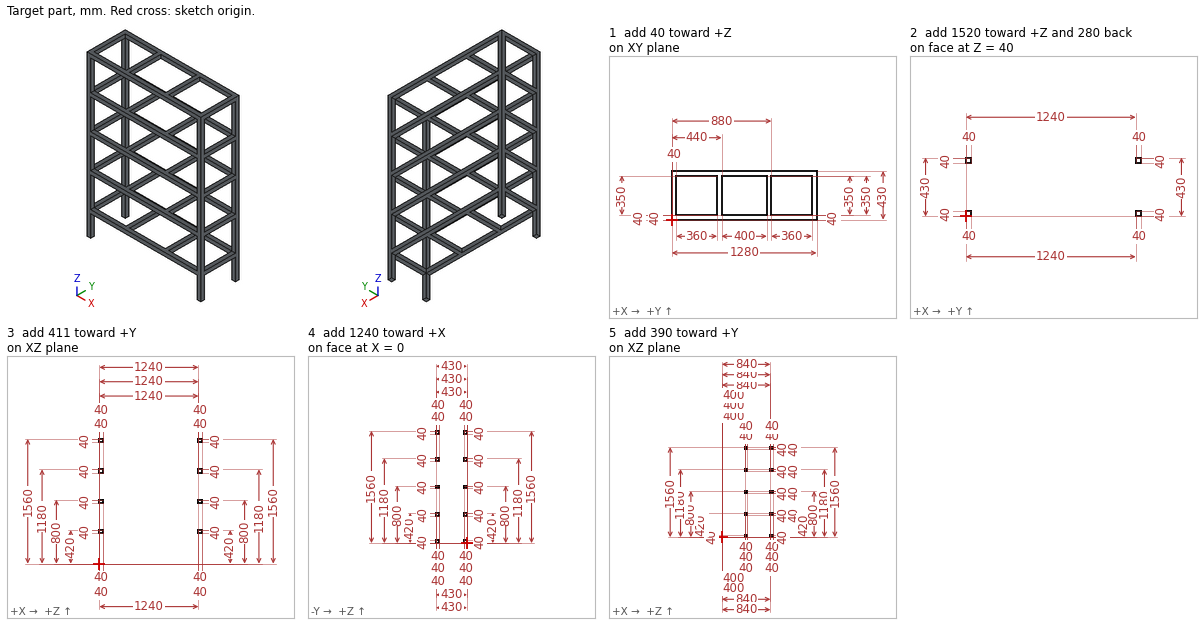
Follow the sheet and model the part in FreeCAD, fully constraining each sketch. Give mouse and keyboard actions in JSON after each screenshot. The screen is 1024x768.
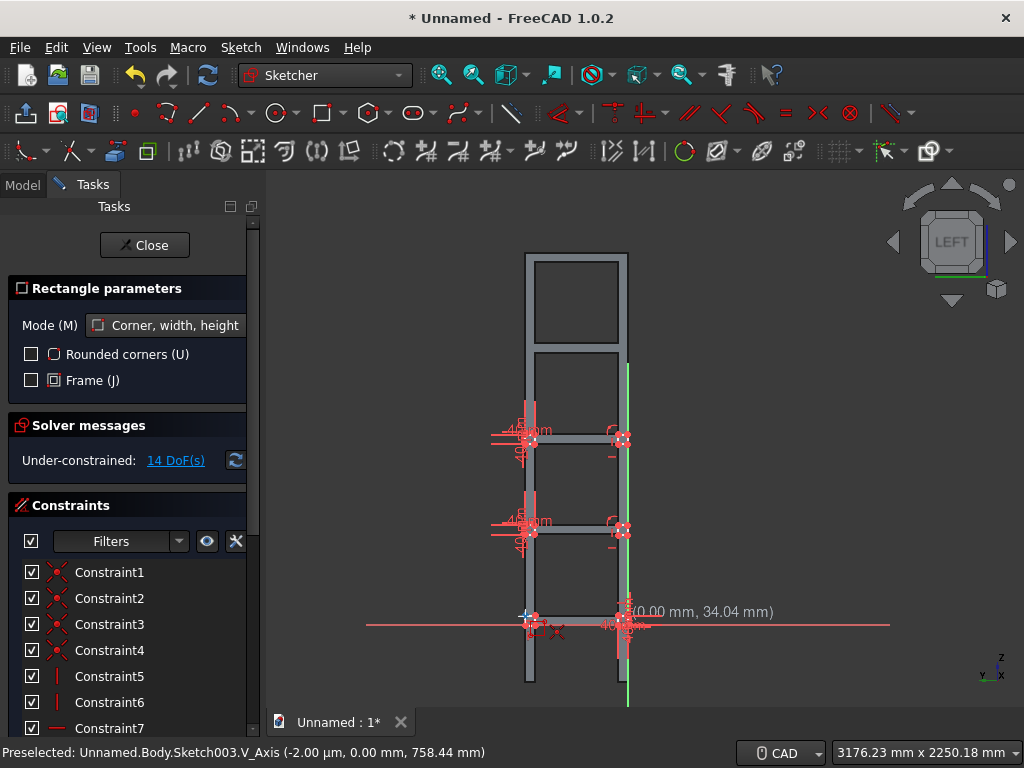
{"action": "scroll", "coordinate": [618, 343], "scroll_direction": "up", "scroll_amount": 3}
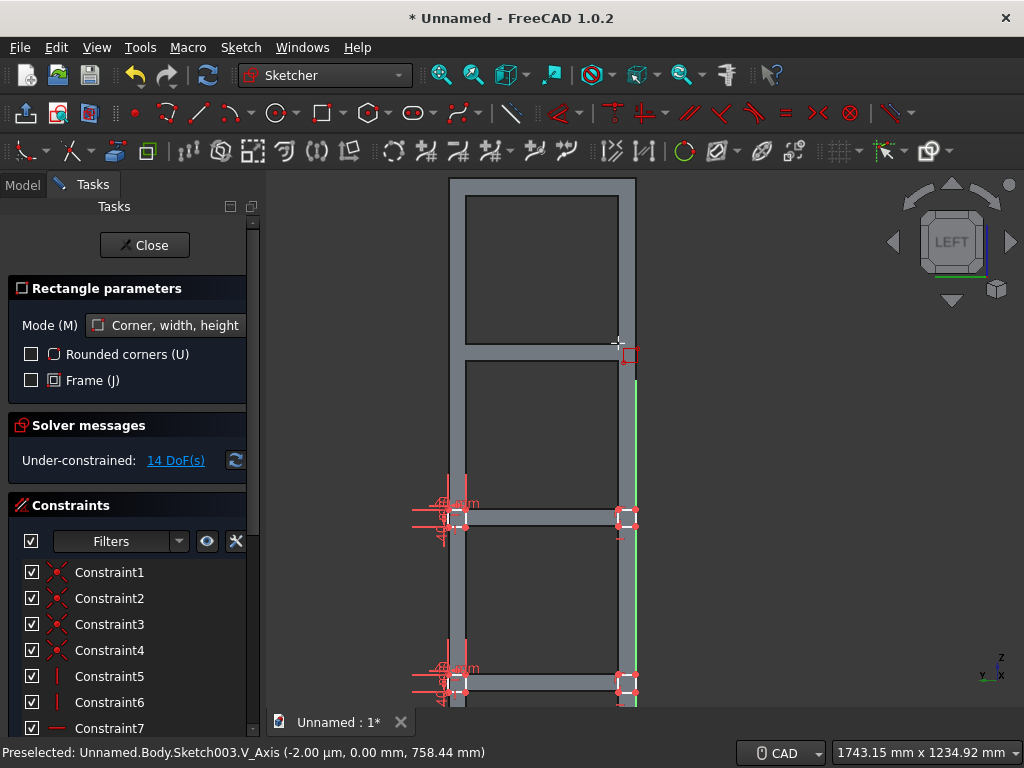
{"action": "left_click", "coordinate": [618, 344]}
{"action": "left_click", "coordinate": [636, 361]}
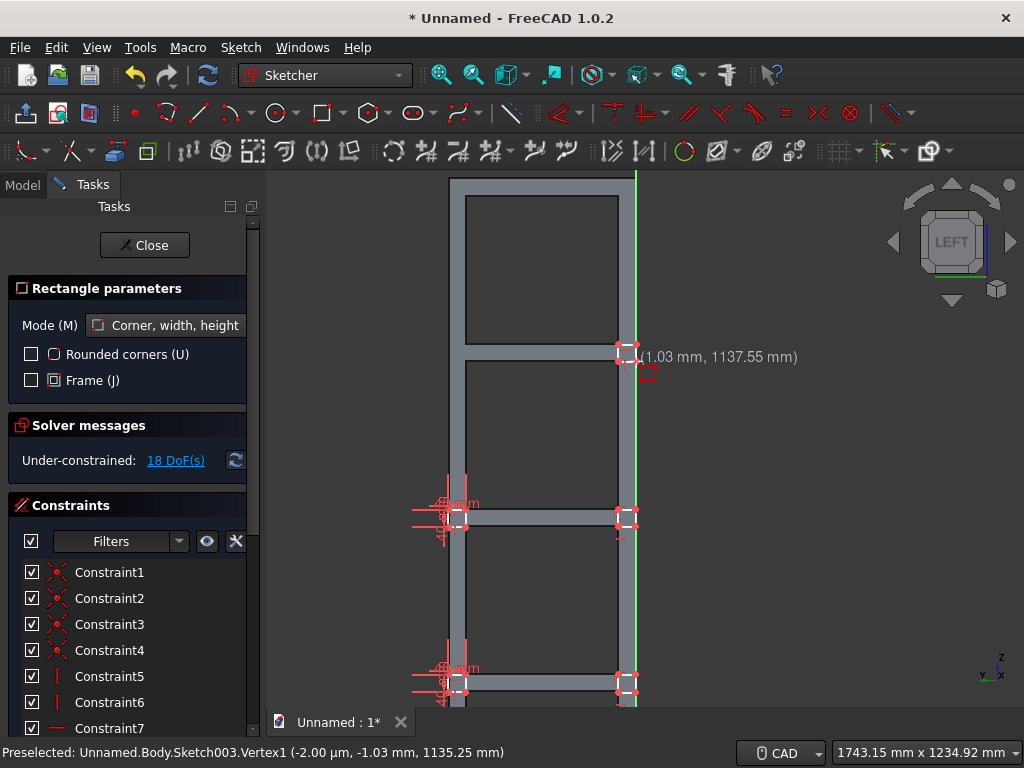
{"action": "left_click", "coordinate": [449, 344]}
{"action": "mouse_move", "coordinate": [466, 361]}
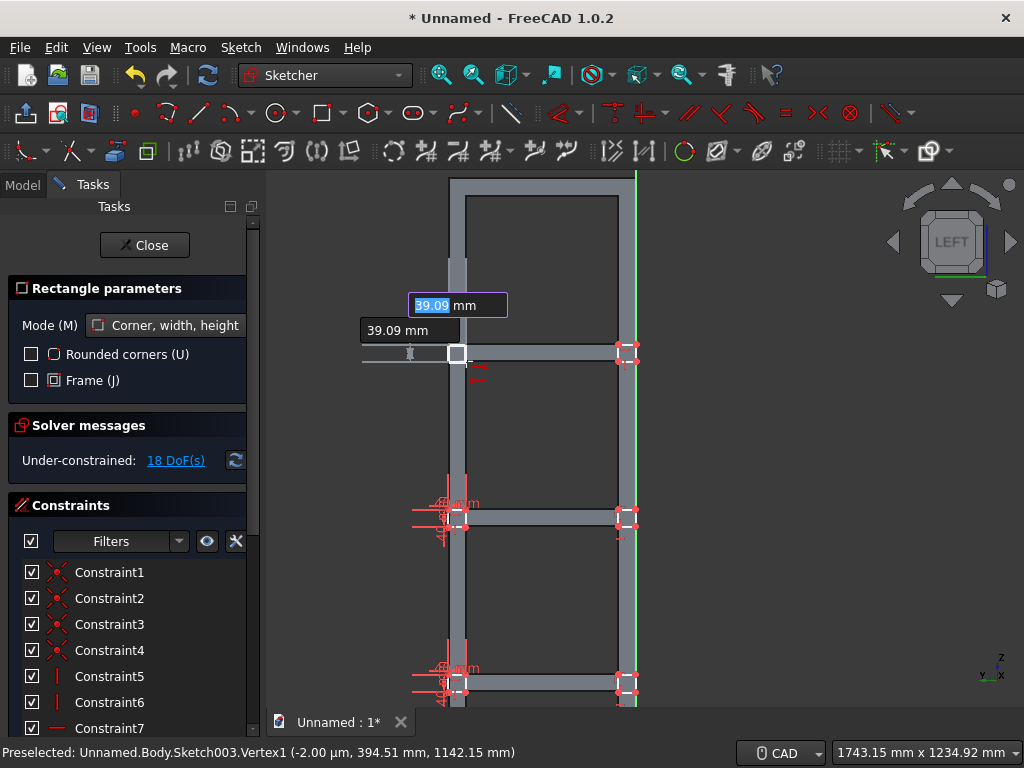
{"action": "type", "text": "40"}
{"action": "key", "text": "Tab"}
{"action": "type", "text": "40"}
{"action": "key", "text": "Return"}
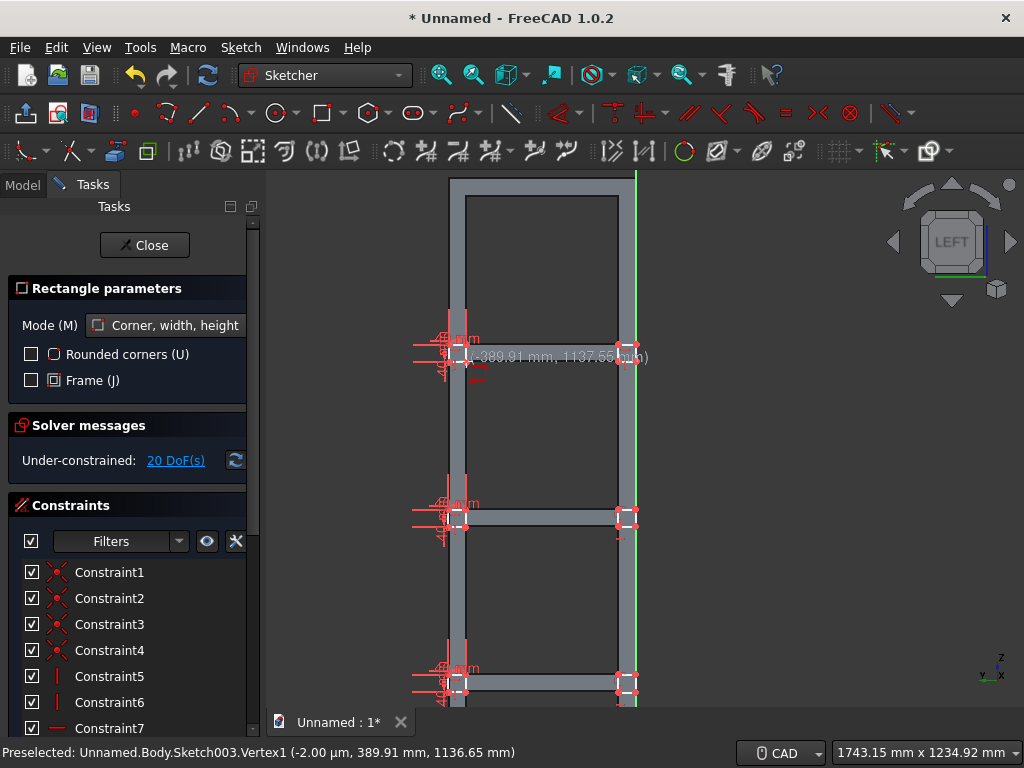
{"action": "scroll", "coordinate": [618, 342], "scroll_direction": "down", "scroll_amount": 3}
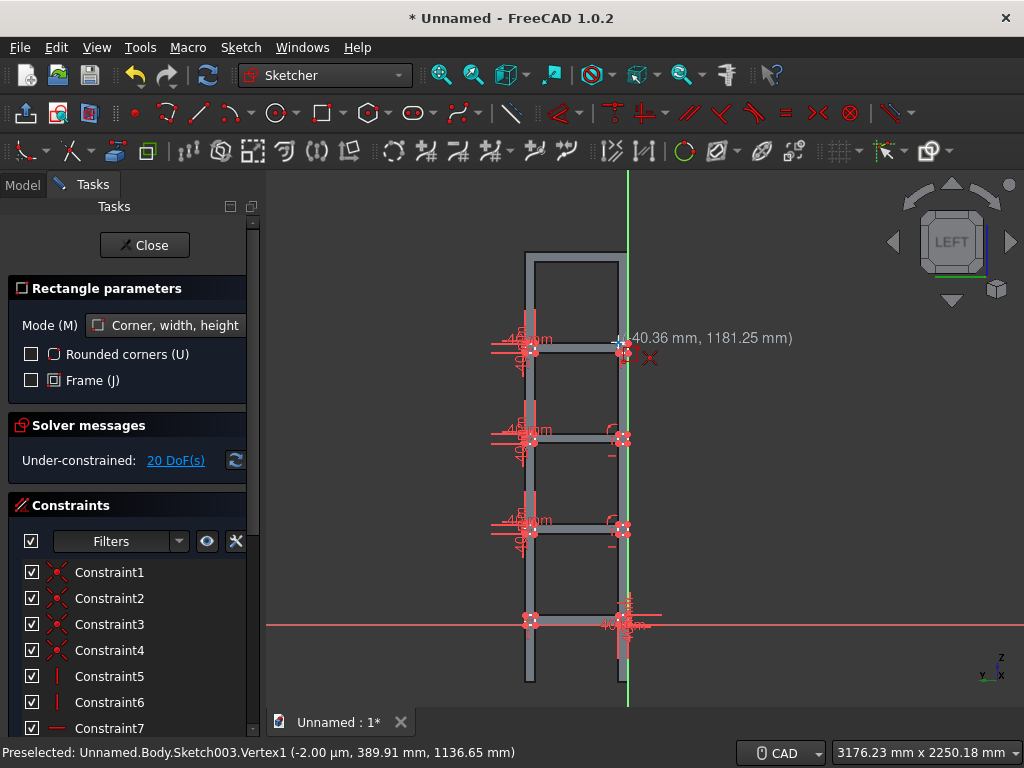
{"action": "scroll", "coordinate": [525, 252], "scroll_direction": "up", "scroll_amount": 3}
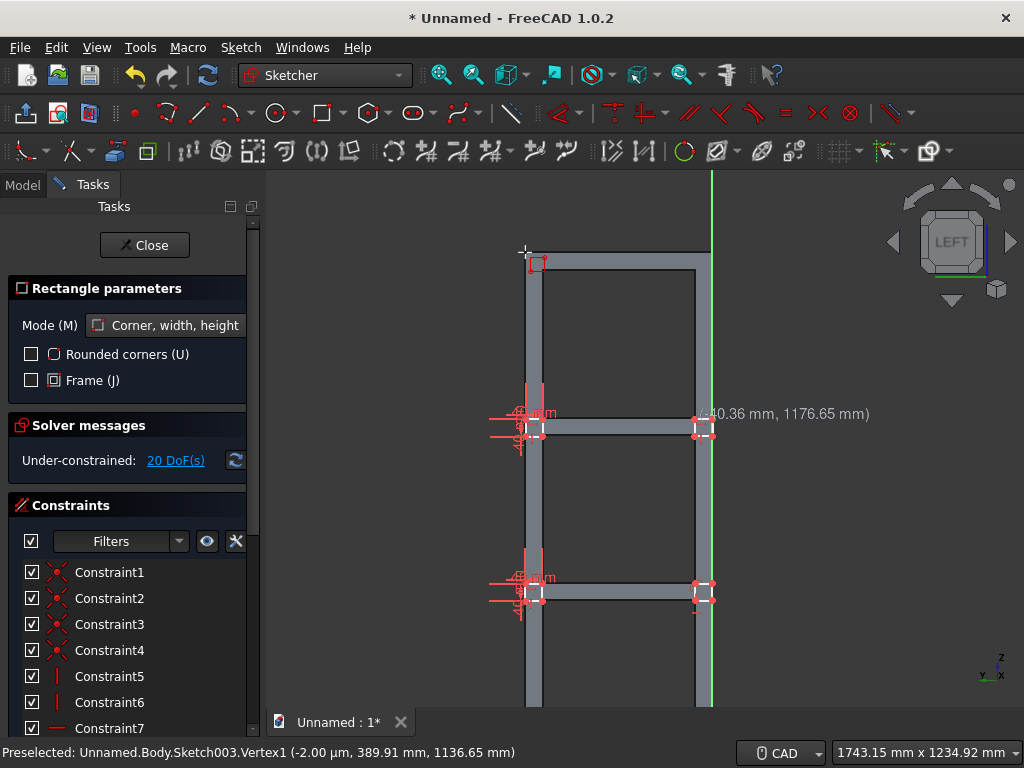
{"action": "left_click", "coordinate": [525, 252]}
{"action": "mouse_move", "coordinate": [543, 270]}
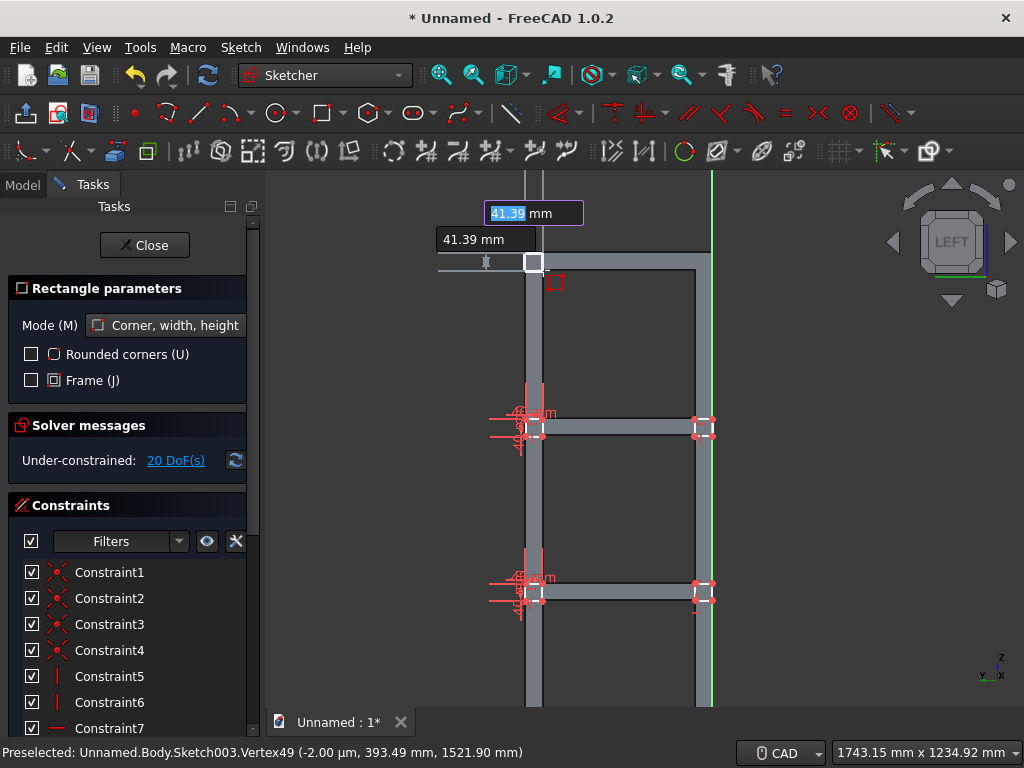
{"action": "type", "text": "40"}
{"action": "key", "text": "Tab"}
{"action": "type", "text": "40"}
{"action": "key", "text": "Return"}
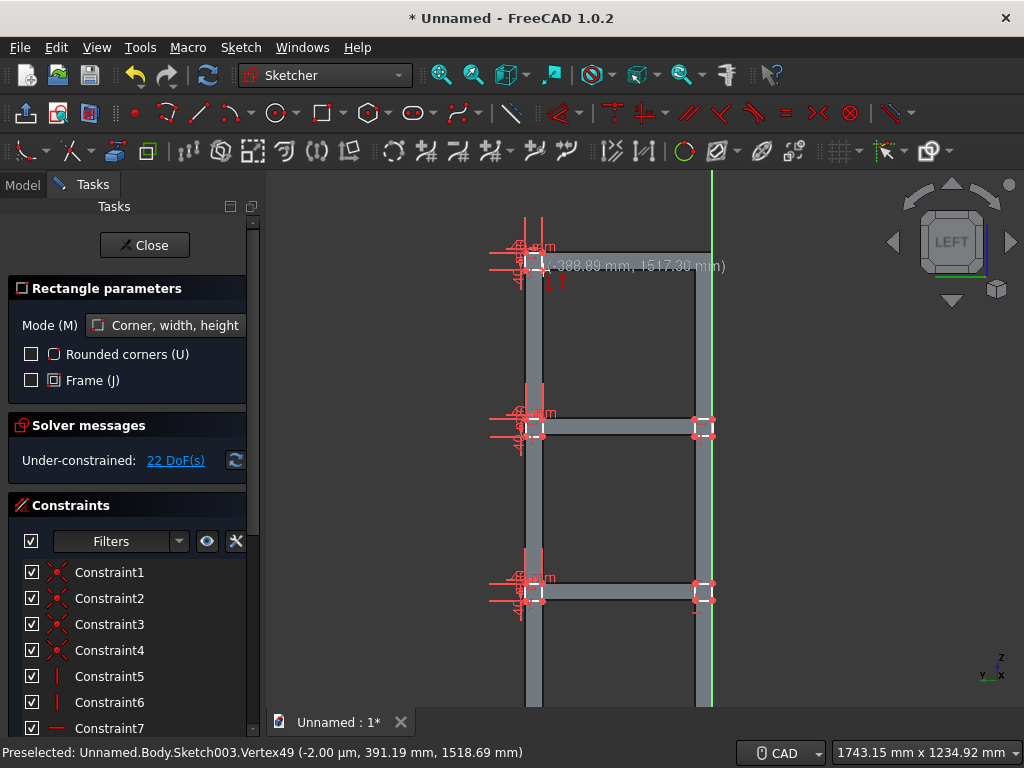
{"action": "left_click", "coordinate": [695, 252]}
{"action": "left_click", "coordinate": [712, 270]}
{"action": "key", "text": "Escape"}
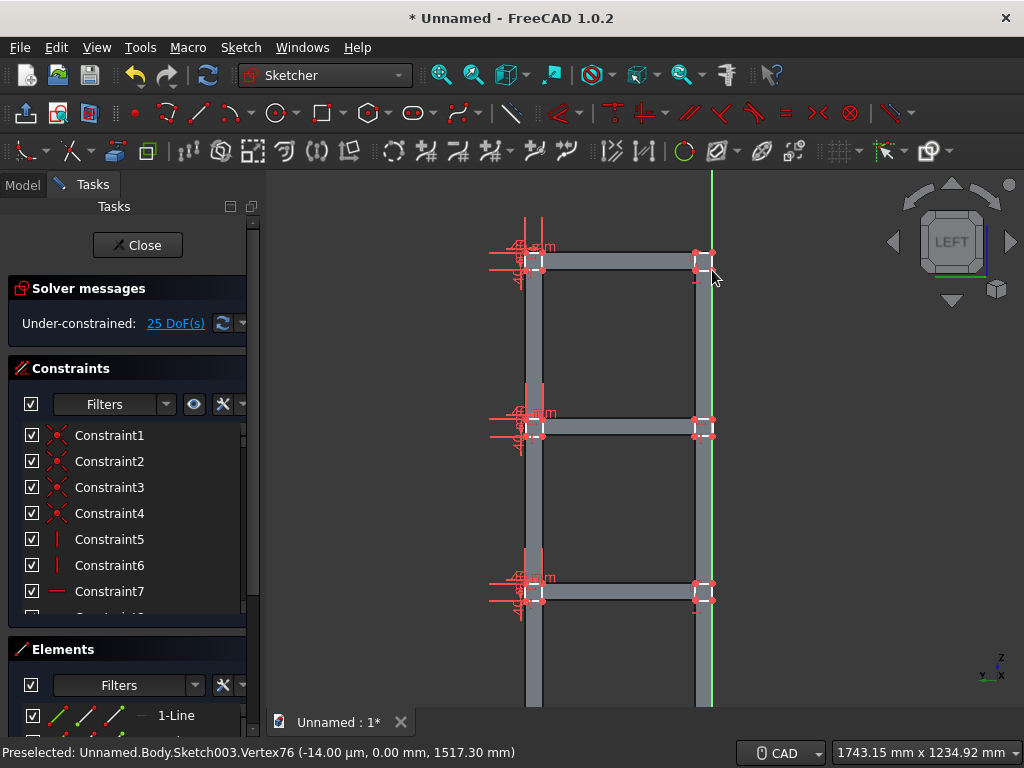
{"action": "scroll", "coordinate": [525, 252], "scroll_direction": "down", "scroll_amount": 3}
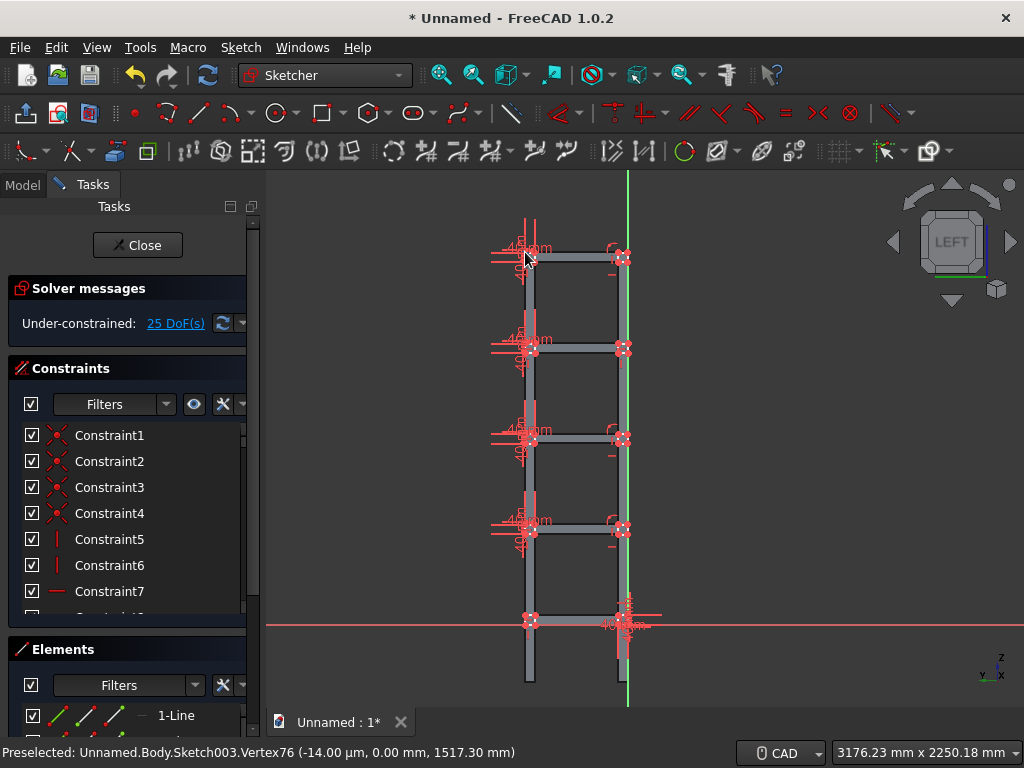
{"action": "scroll", "coordinate": [525, 625], "scroll_direction": "up", "scroll_amount": 2}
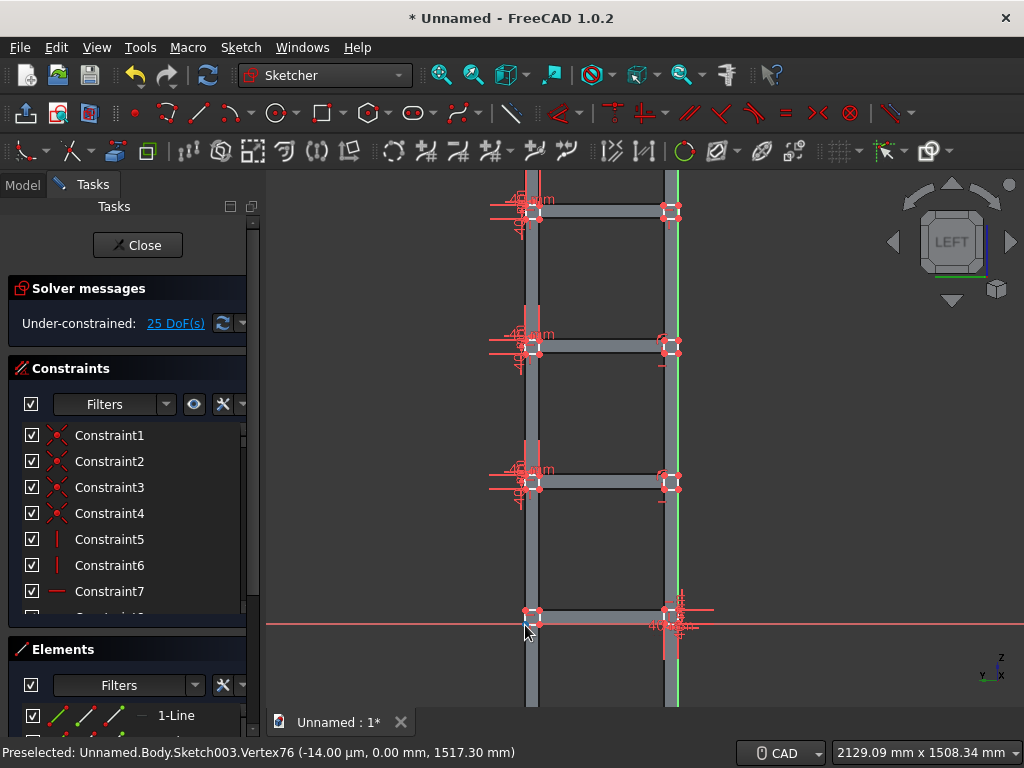
{"action": "left_click", "coordinate": [525, 625]}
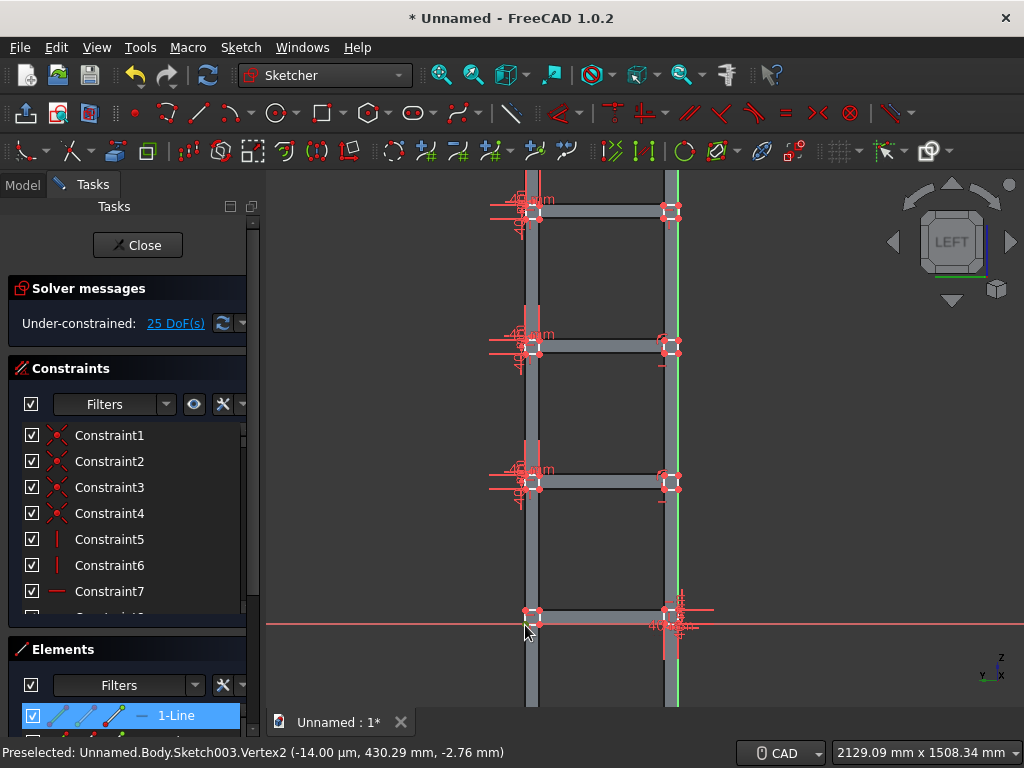
{"action": "left_click", "coordinate": [334, 624]}